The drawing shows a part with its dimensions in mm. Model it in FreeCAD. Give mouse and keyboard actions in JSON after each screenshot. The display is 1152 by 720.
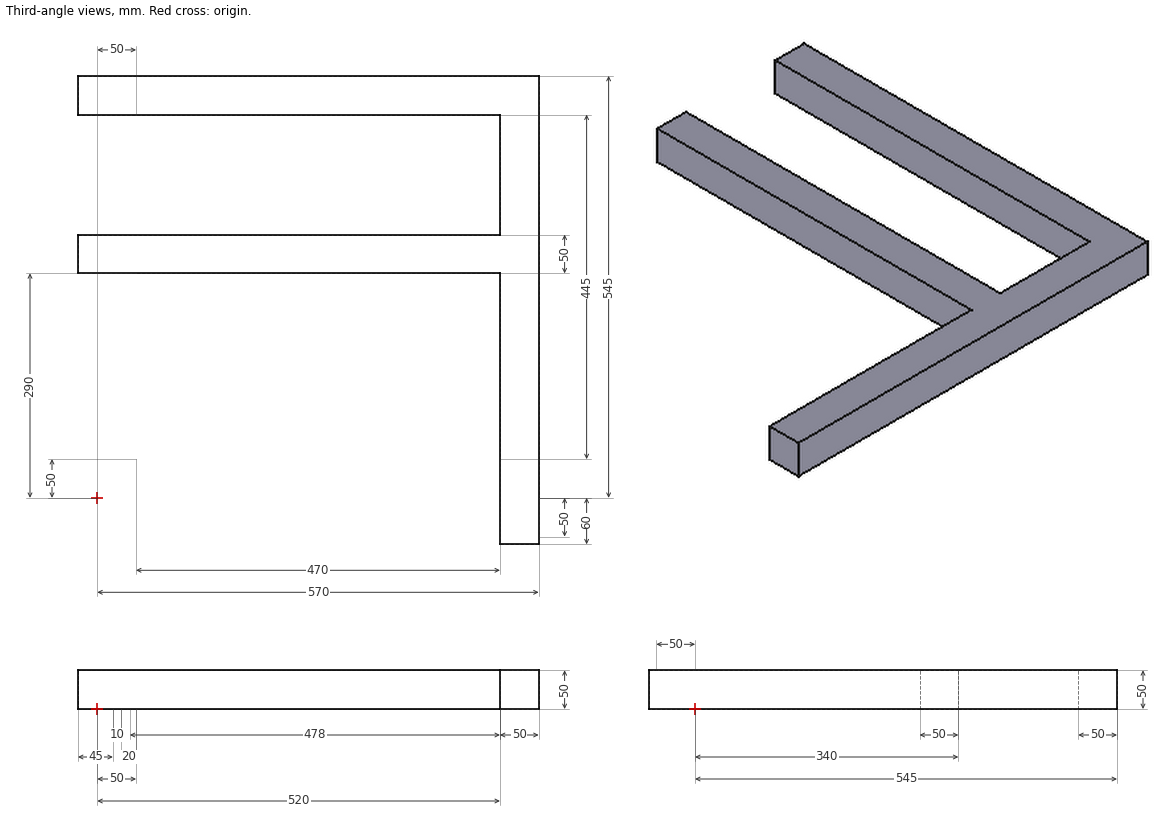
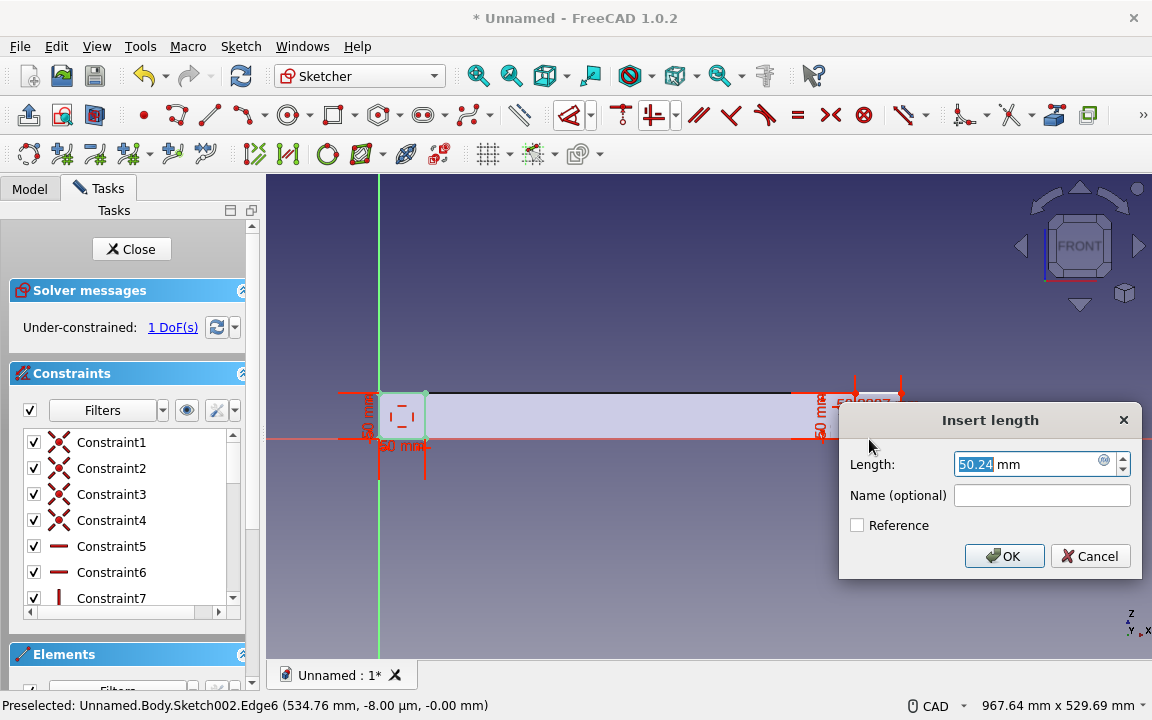
{"action": "type", "text": "50"}
{"action": "key", "text": "Return"}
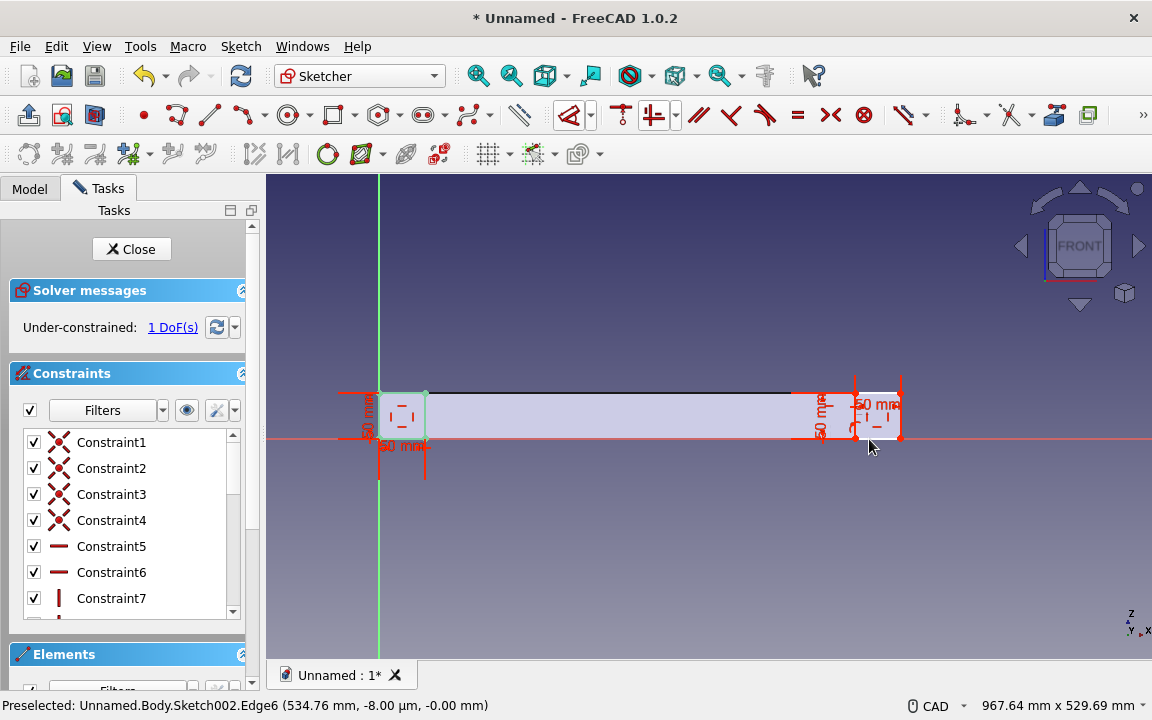
{"action": "left_click", "coordinate": [855, 393]}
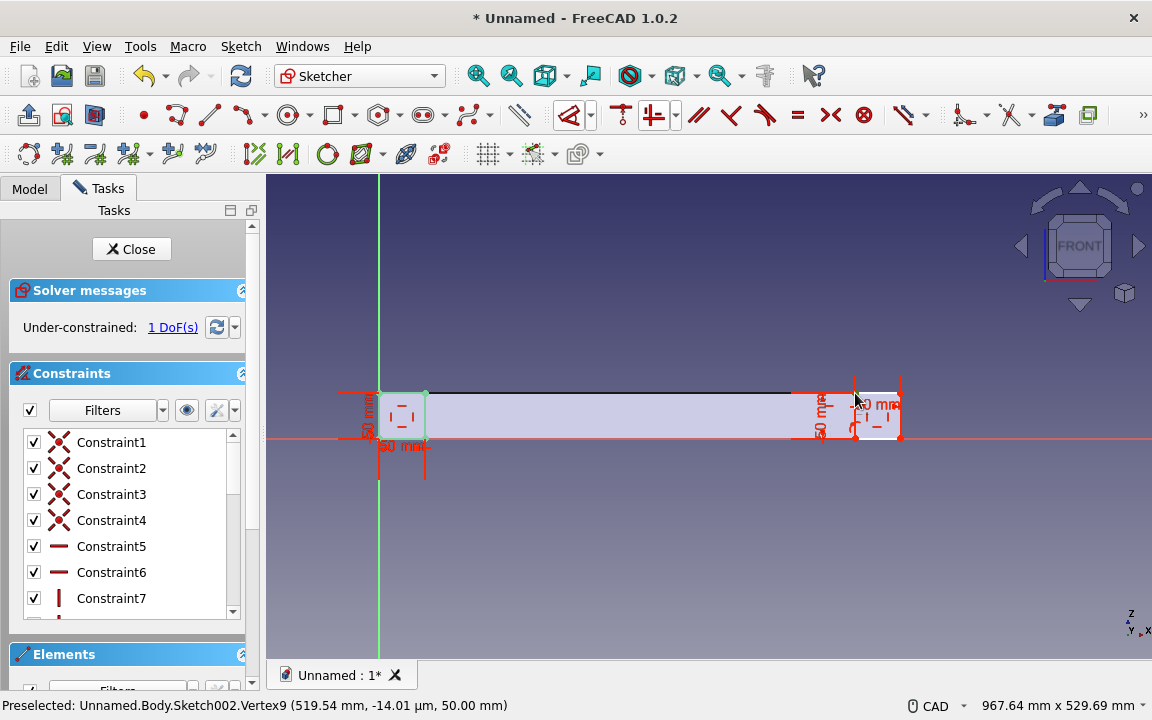
{"action": "key", "text": "l"}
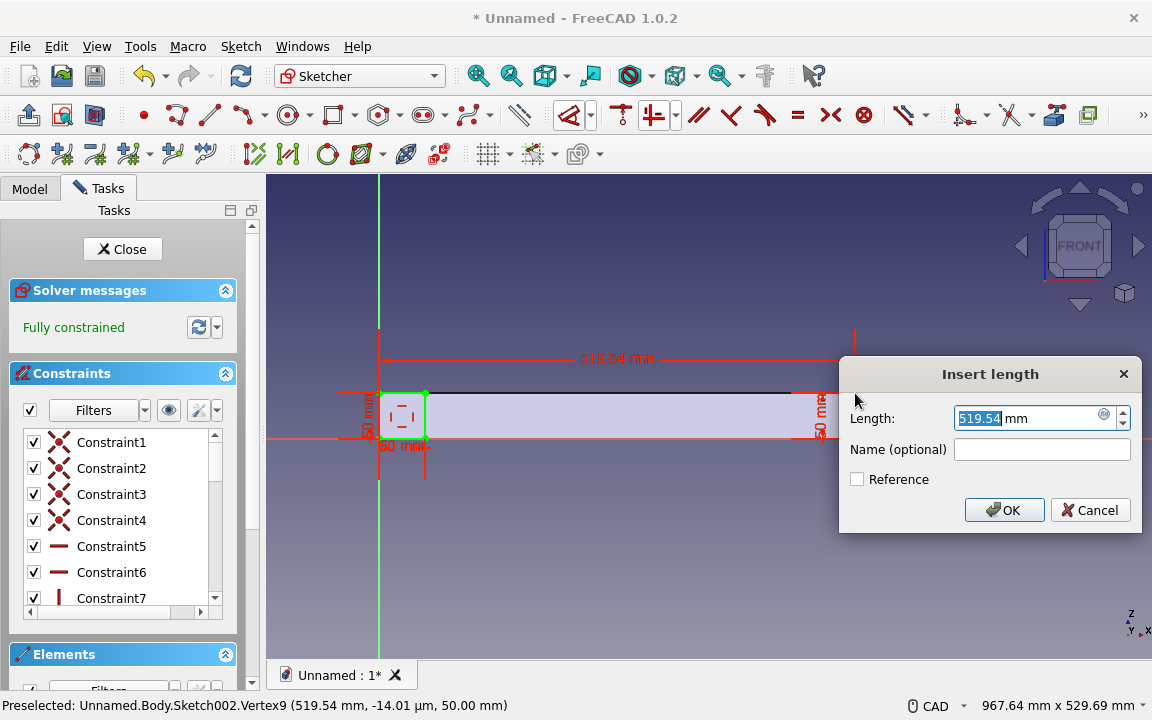
{"action": "type", "text": "520"}
{"action": "key", "text": "Return"}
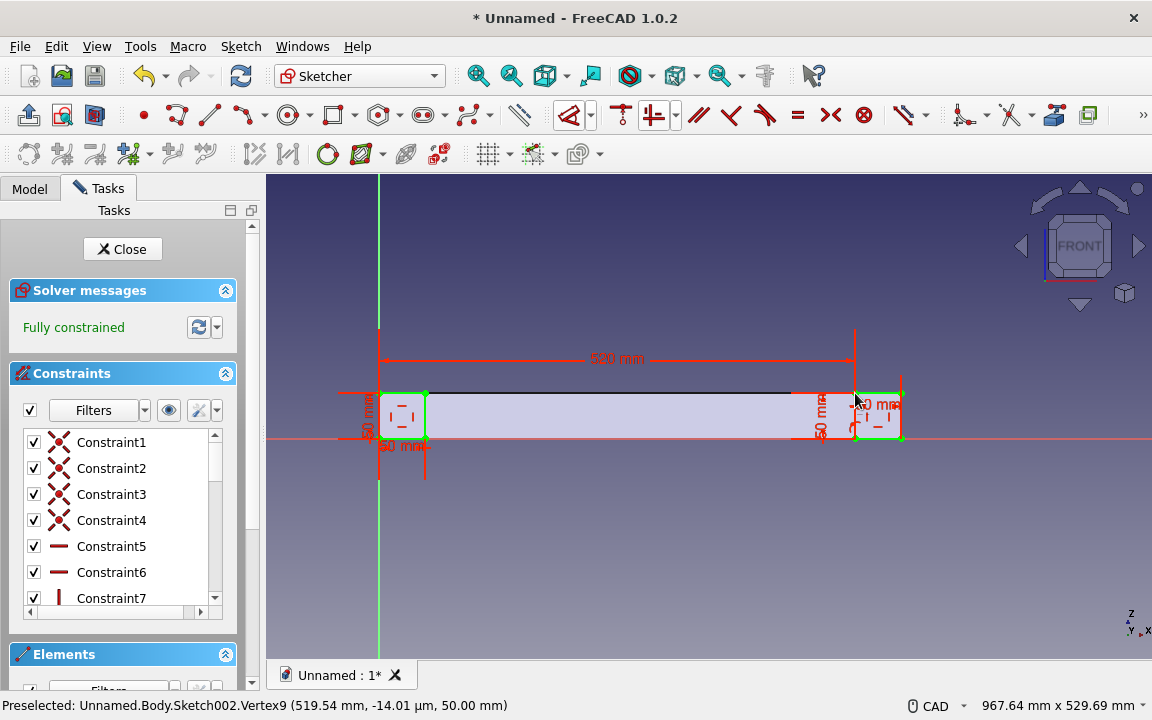
{"action": "left_click", "coordinate": [123, 249]}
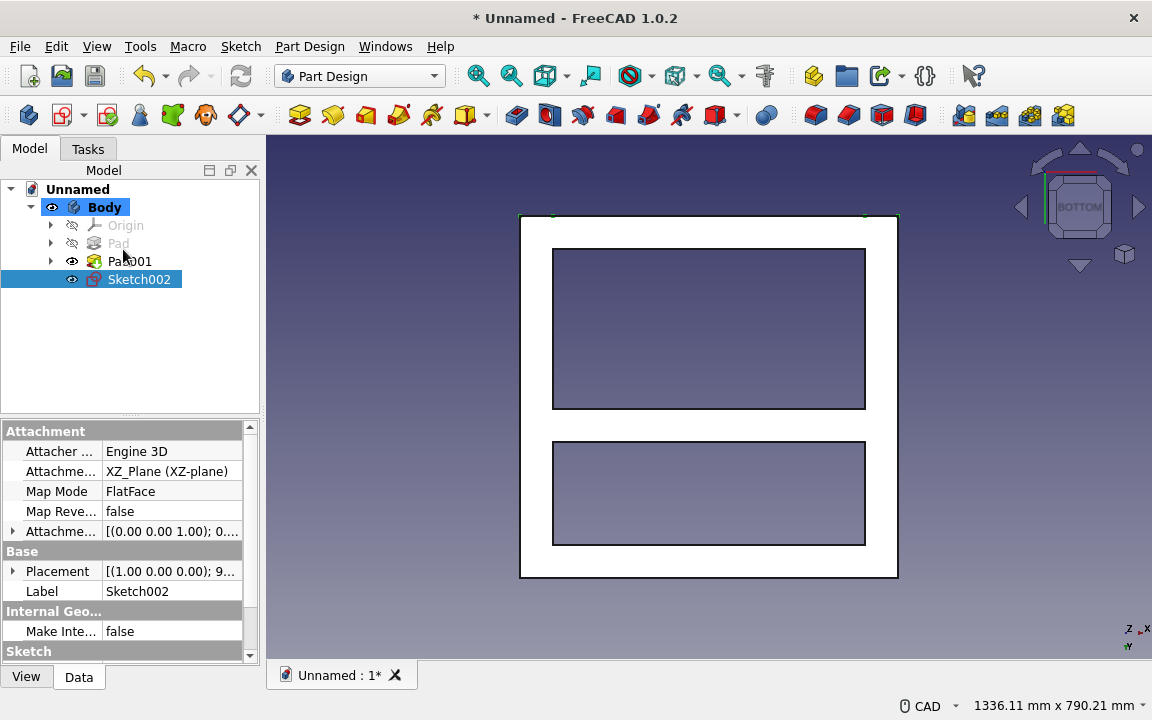
{"action": "left_click", "coordinate": [300, 116]}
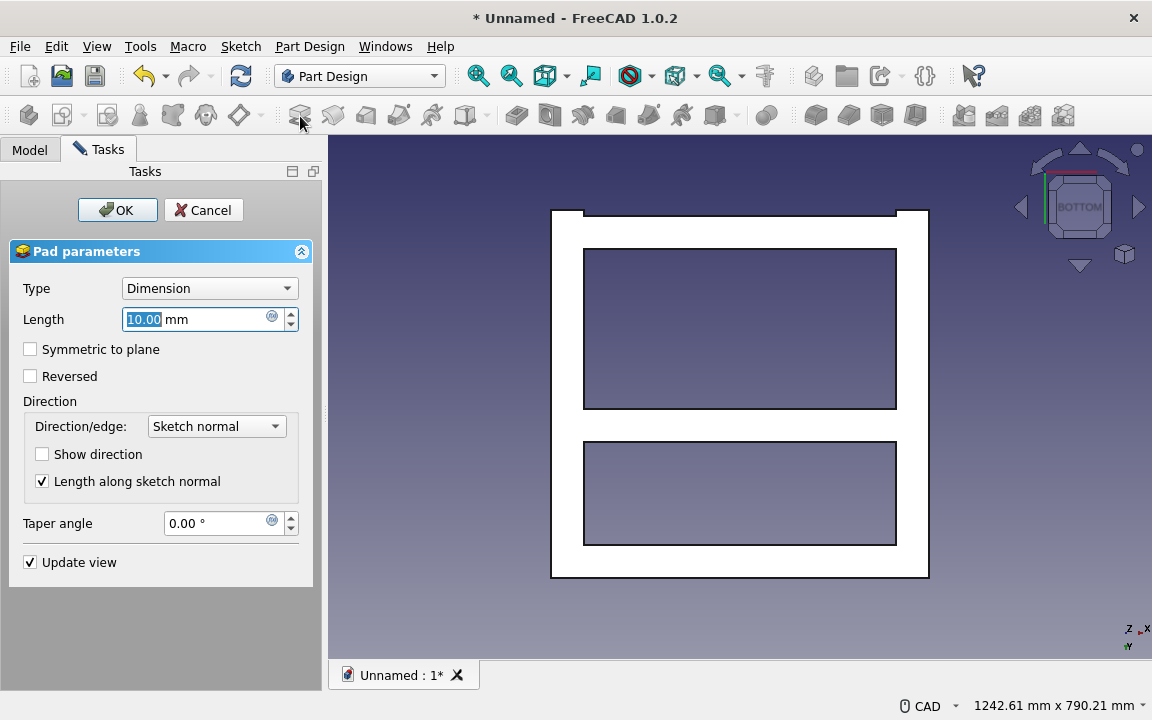
{"action": "type", "text": "50"}
{"action": "key", "text": "Tab"}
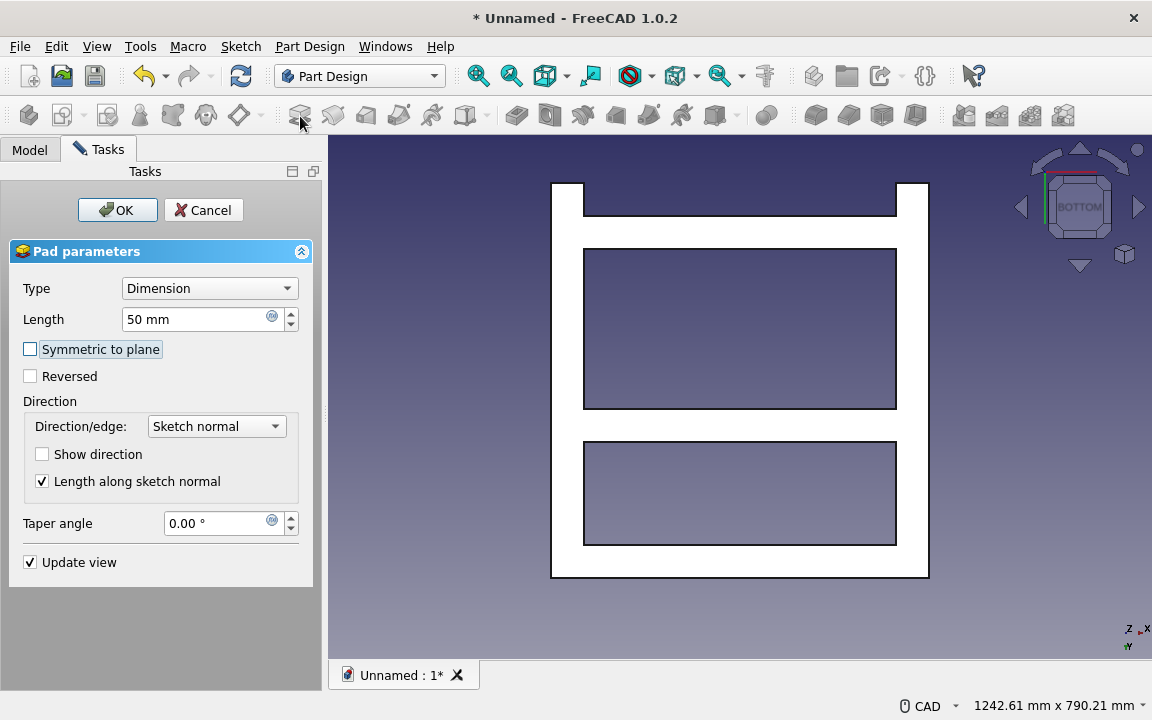
{"action": "left_click", "coordinate": [118, 210]}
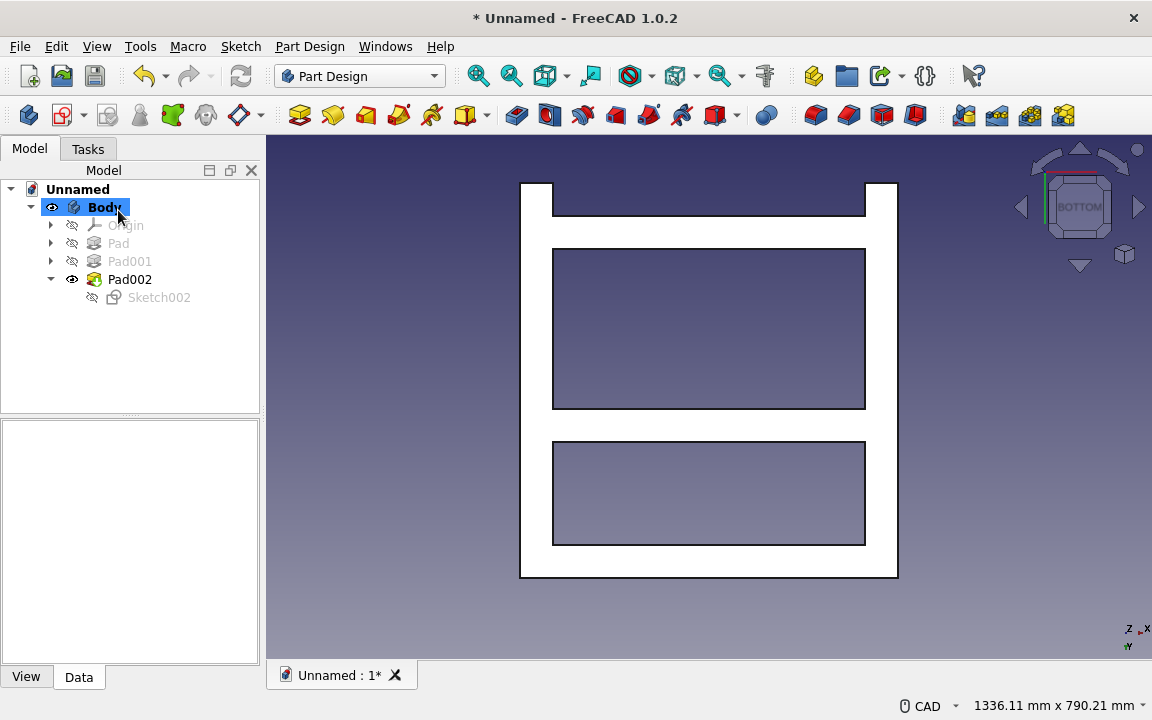
{"action": "key", "text": "0"}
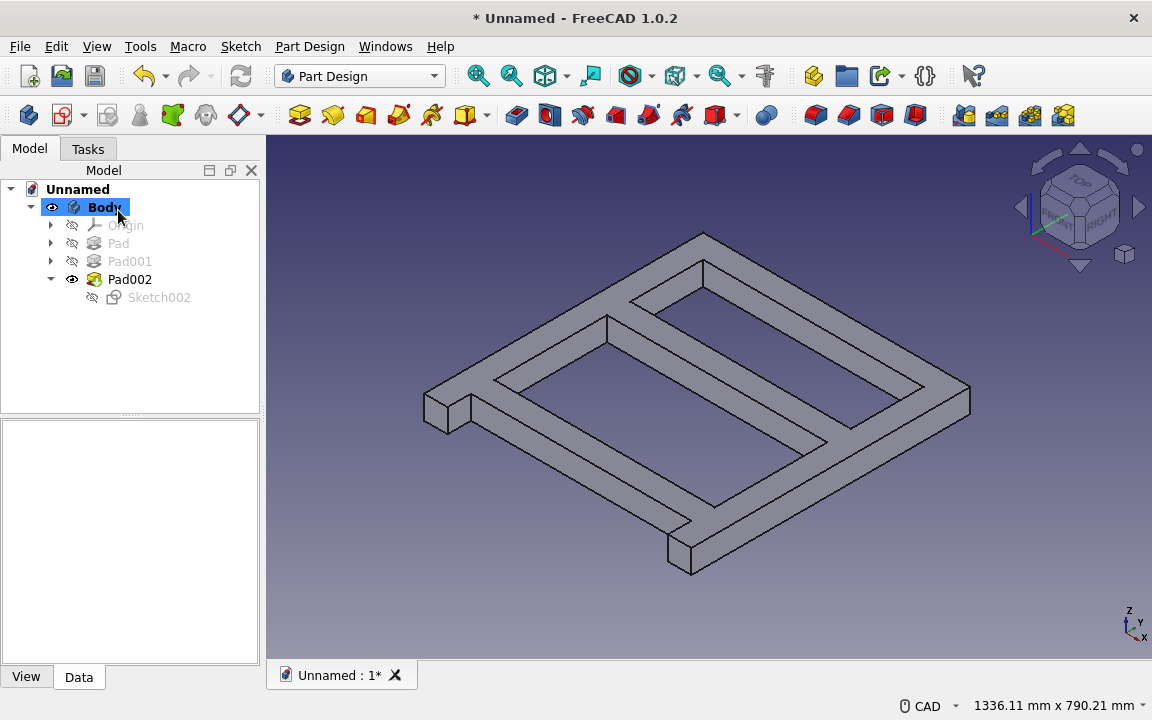
{"action": "left_click", "coordinate": [931, 386]}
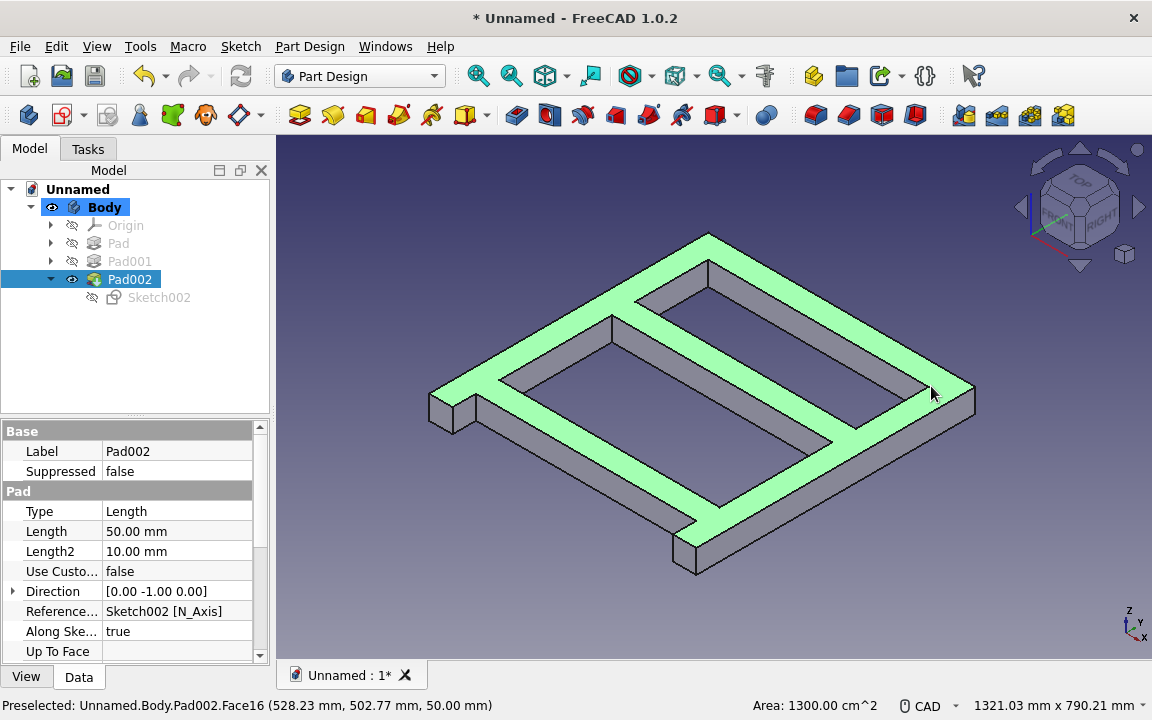
{"action": "left_click", "coordinate": [62, 116]}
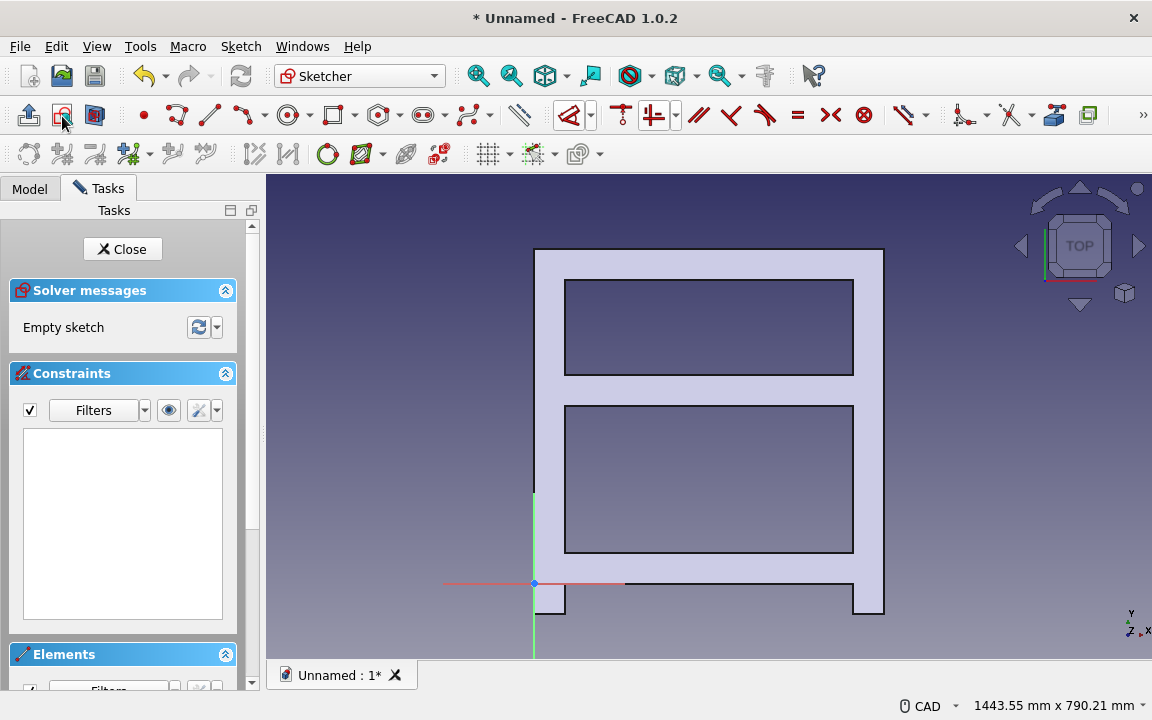
{"action": "scroll", "coordinate": [802, 631], "scroll_direction": "up", "scroll_amount": 2}